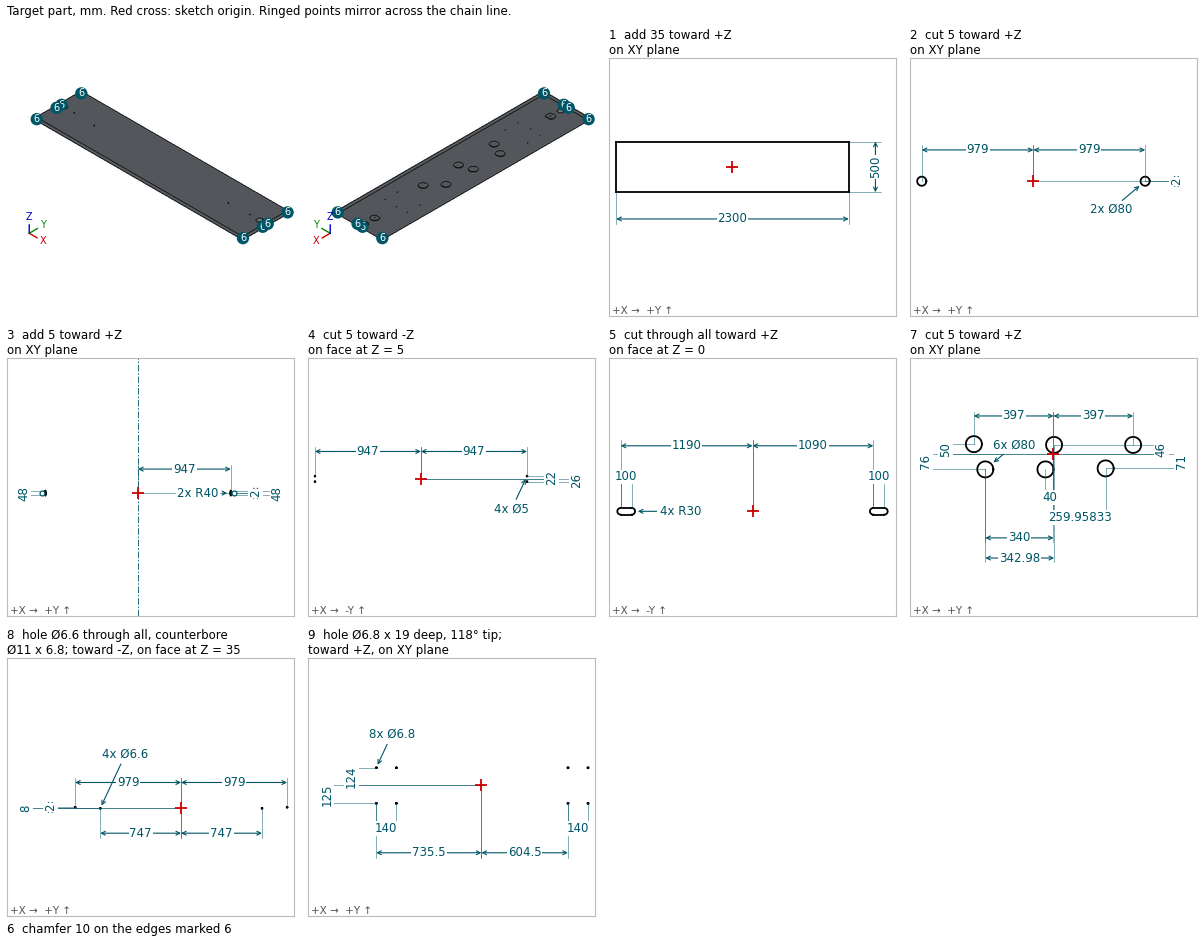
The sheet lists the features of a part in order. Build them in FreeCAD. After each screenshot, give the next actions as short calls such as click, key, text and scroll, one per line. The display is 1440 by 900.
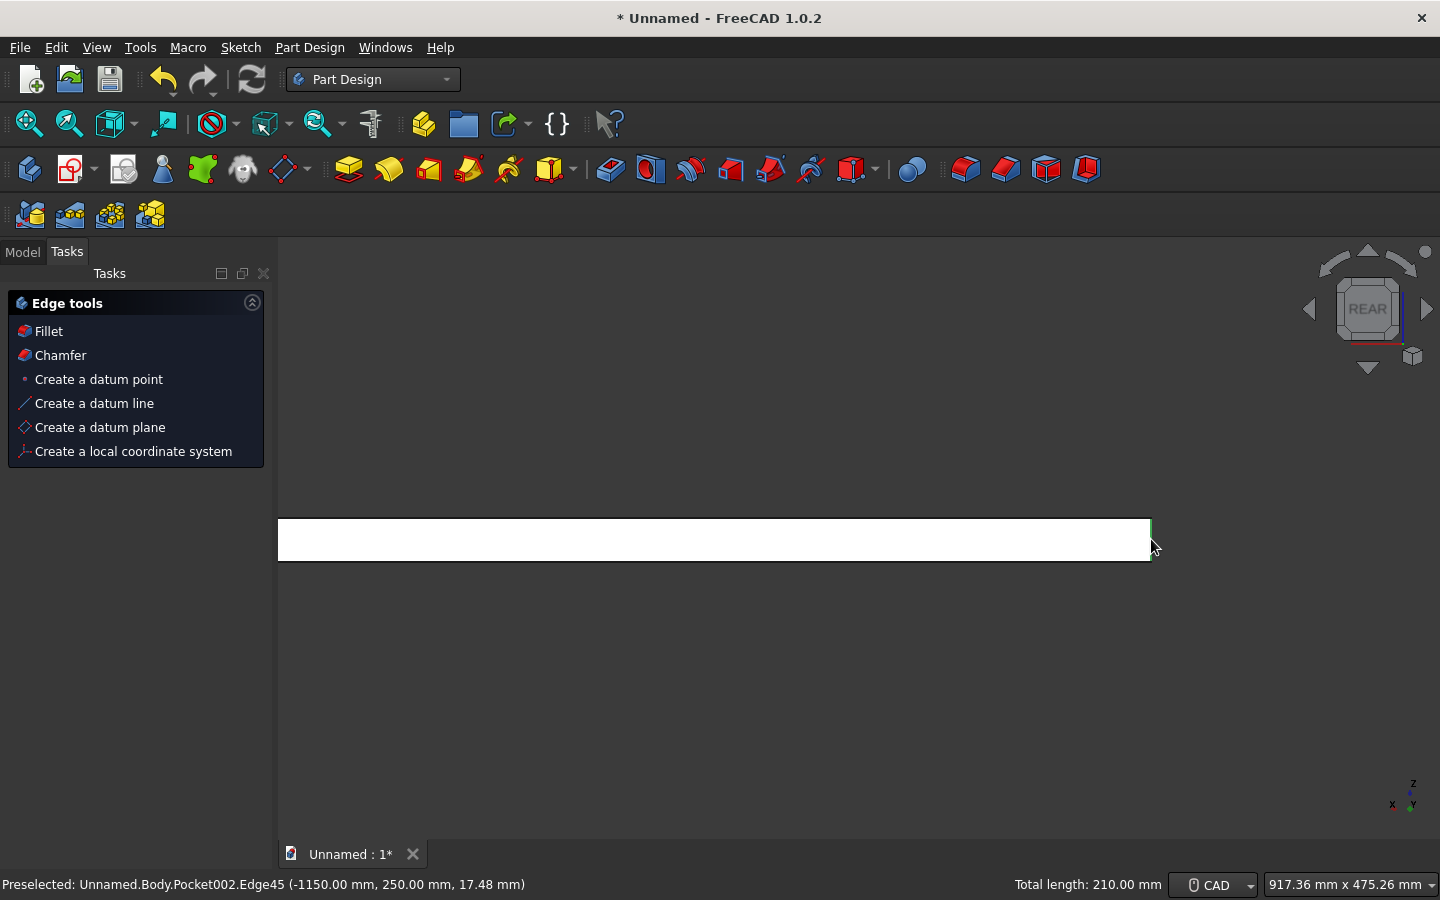
click(30, 124)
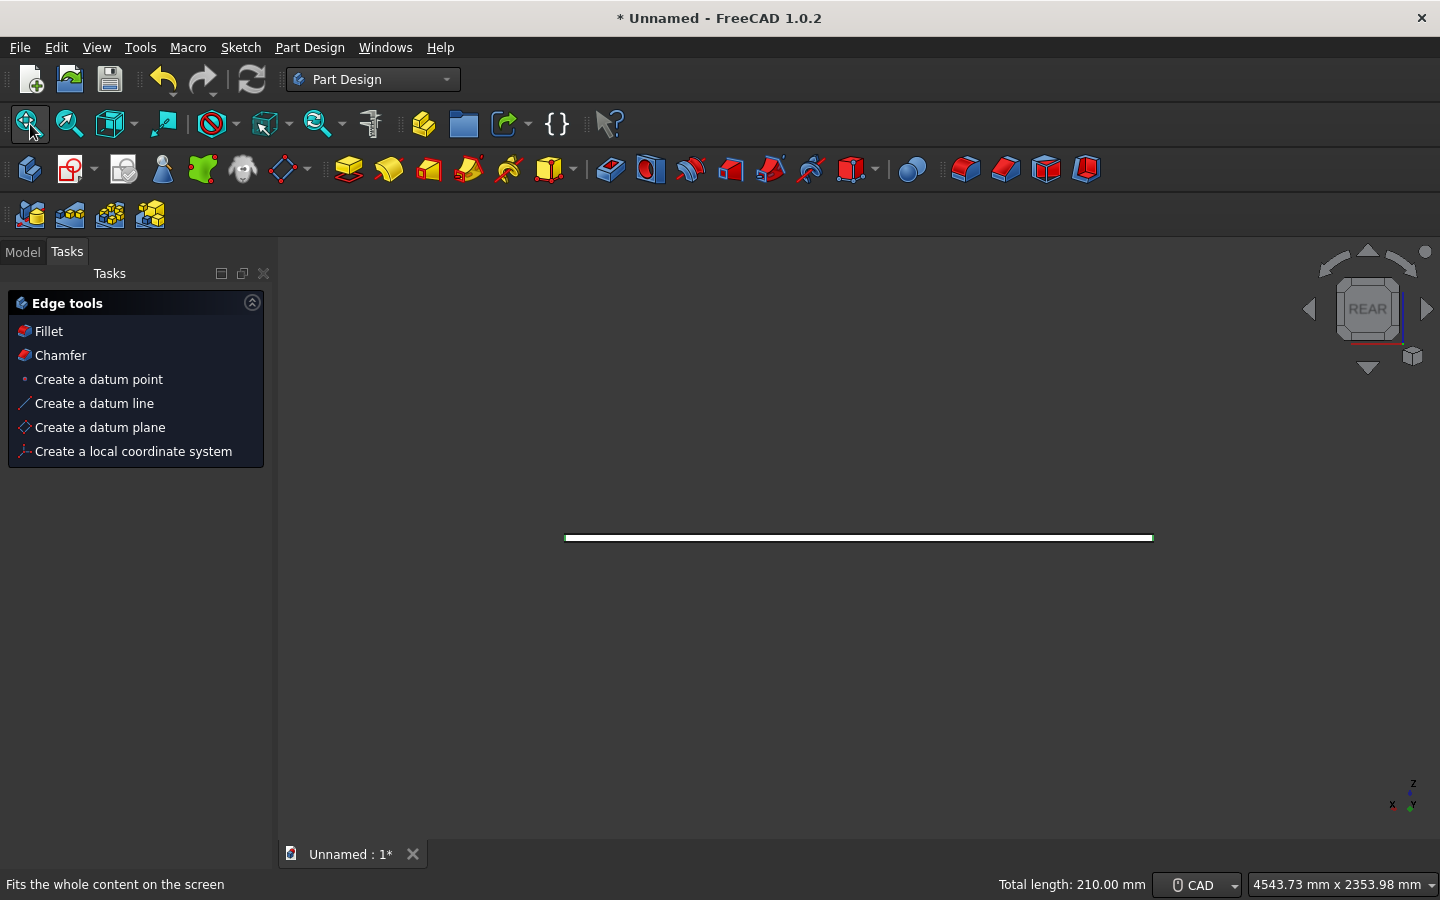
key(6)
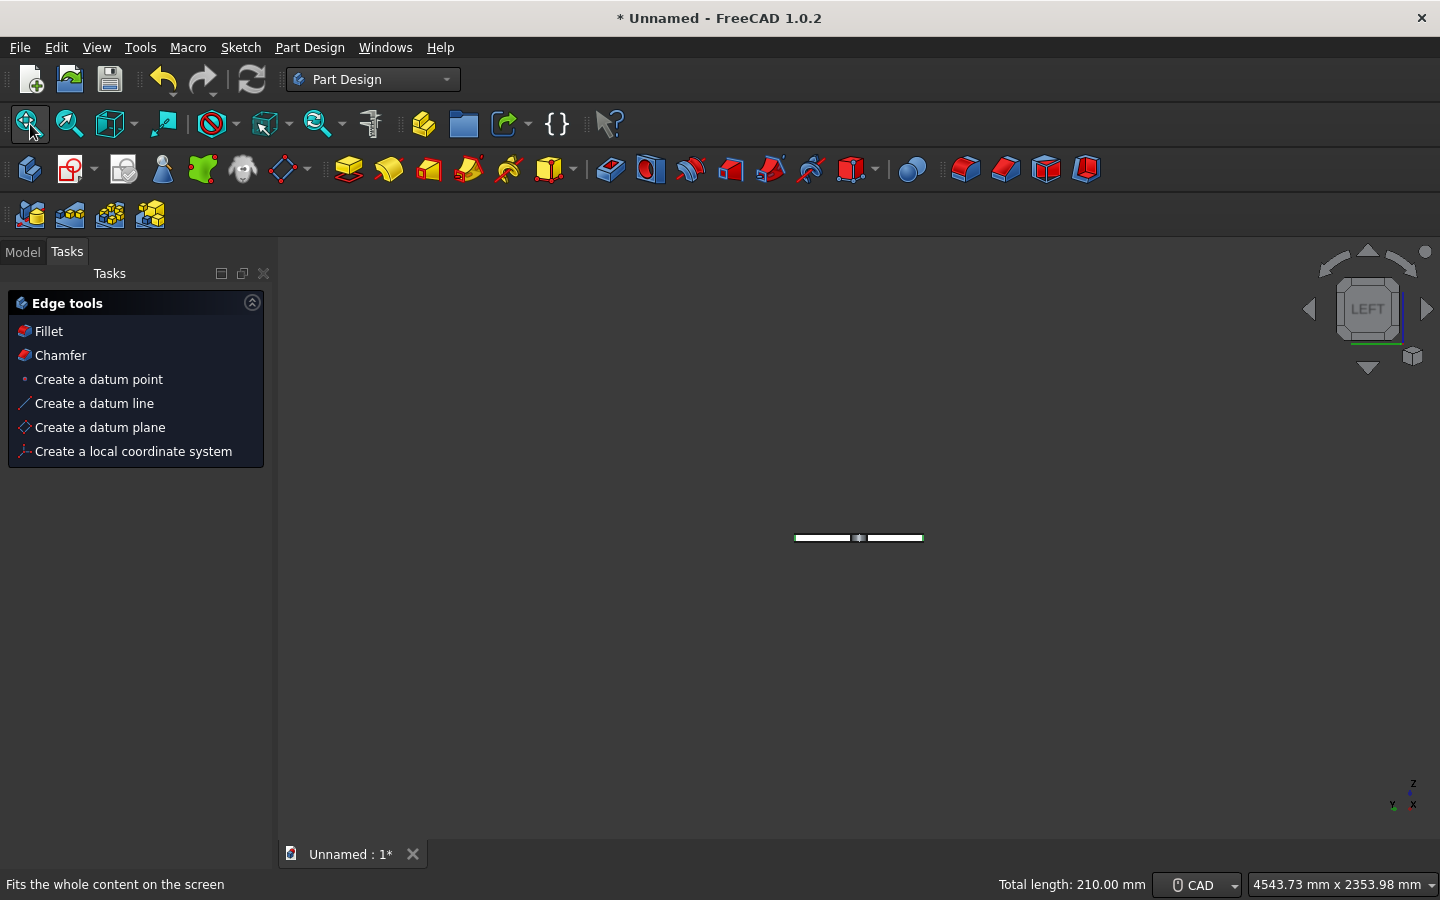
click(30, 124)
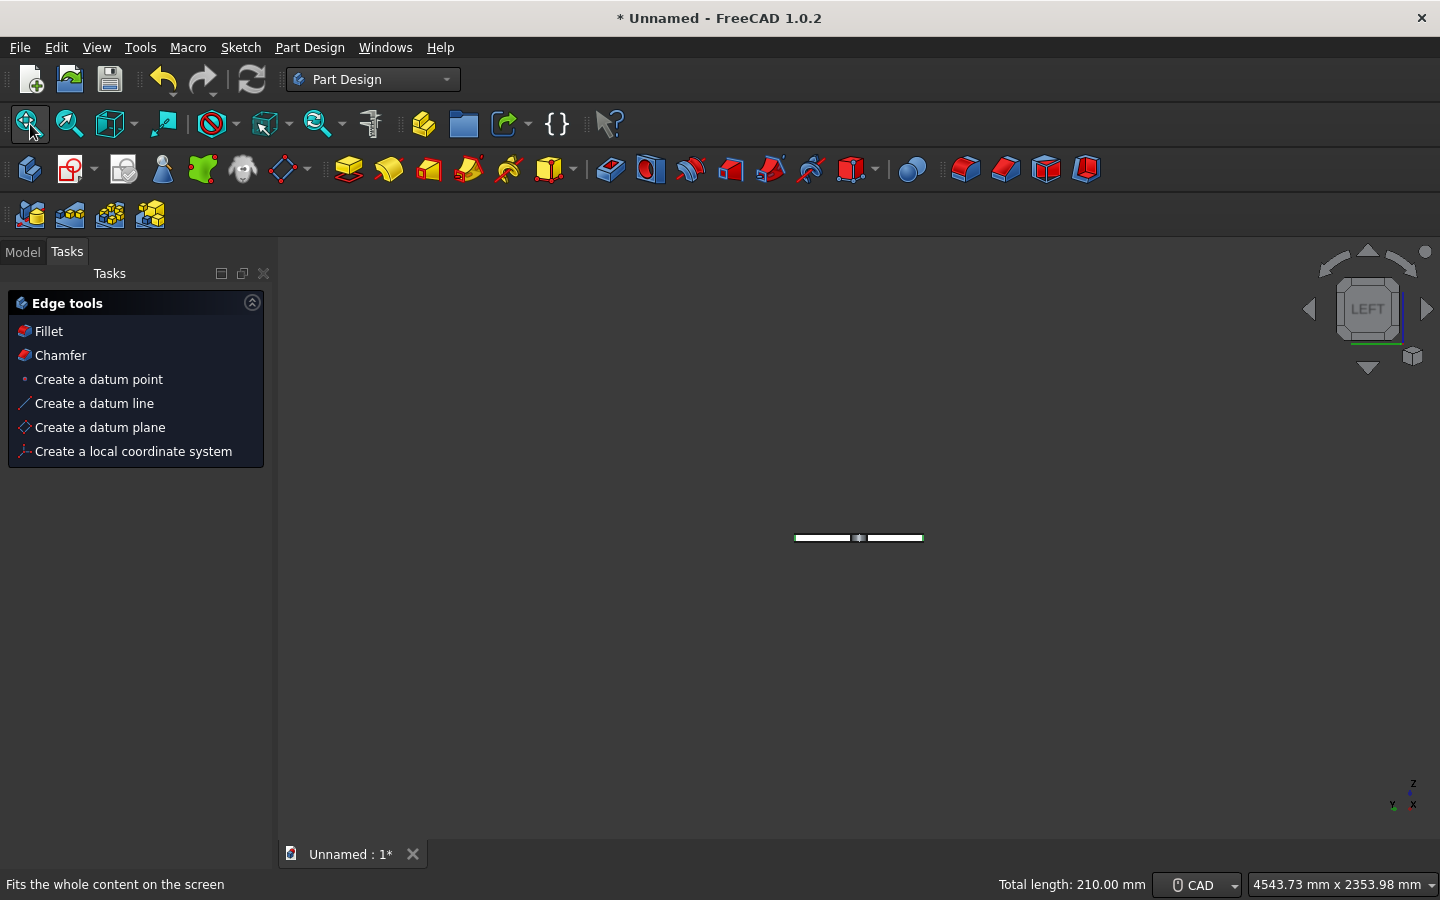
scroll(851, 537, up, 8)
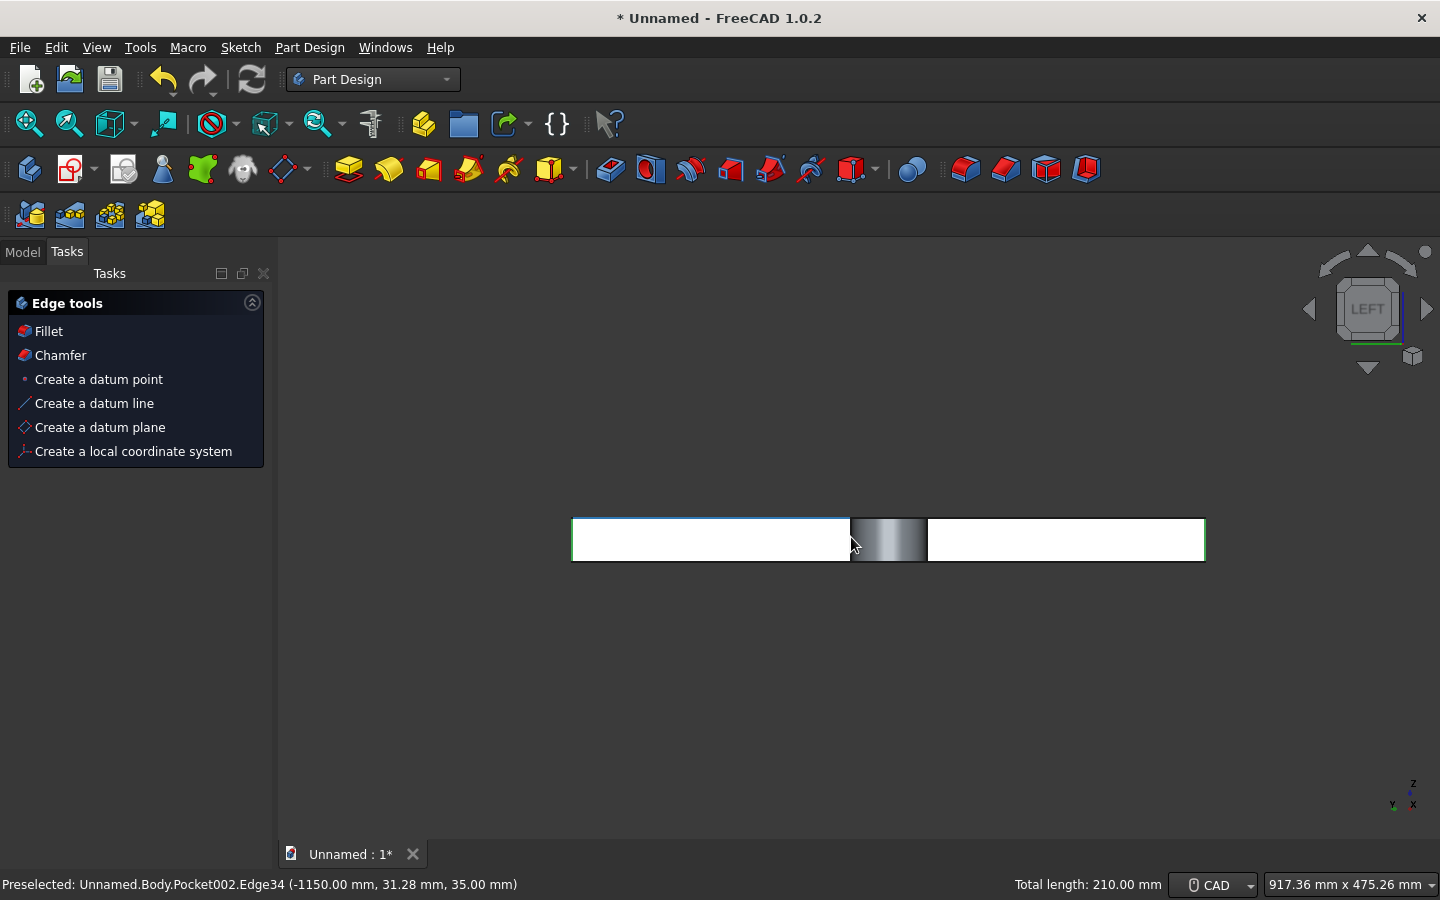
click(851, 539, ctrl)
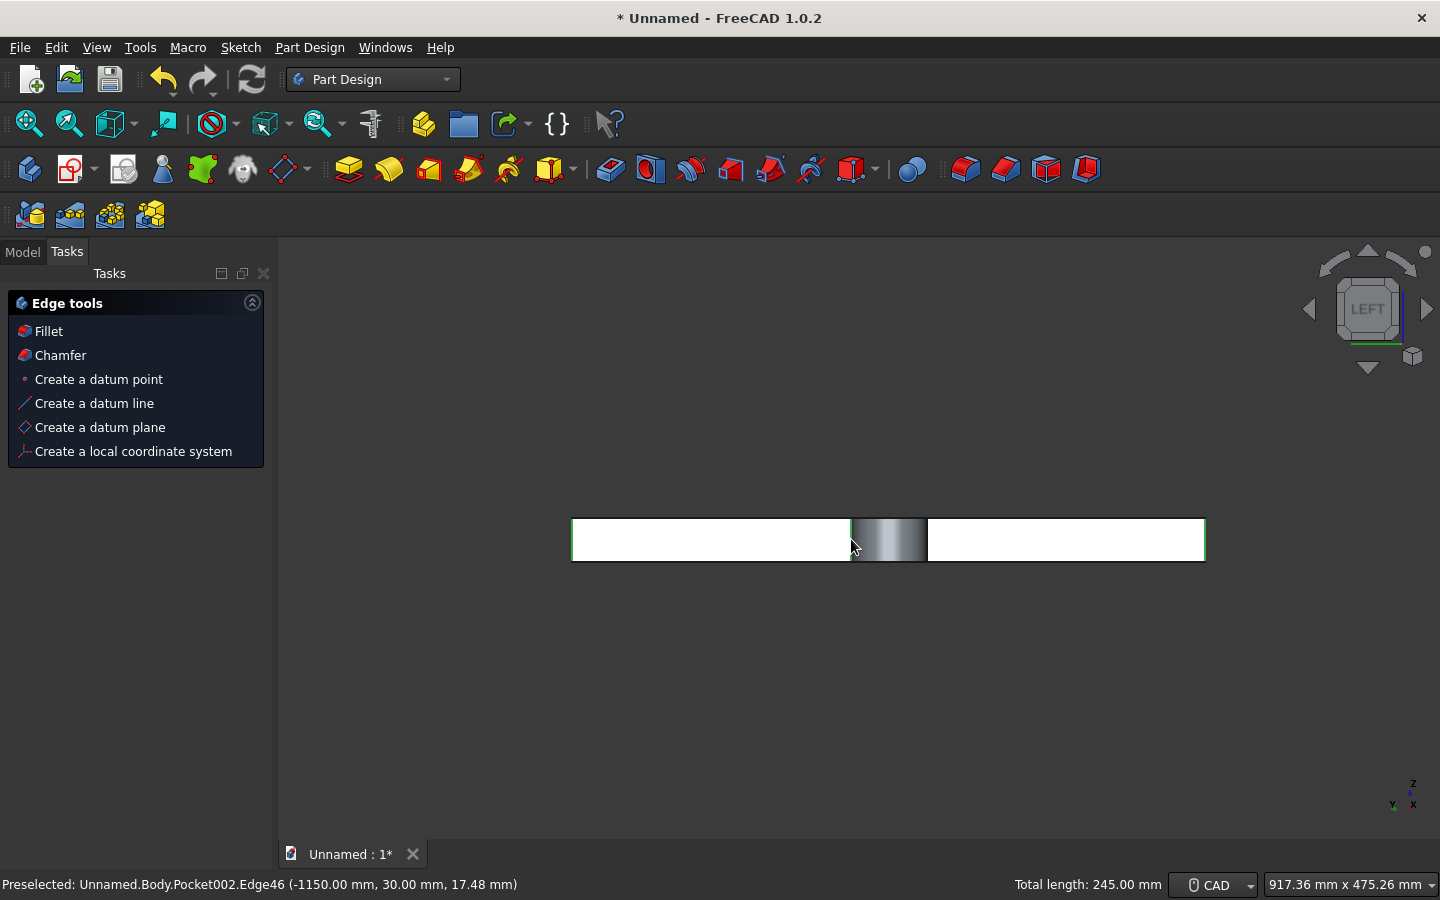
click(927, 539, ctrl)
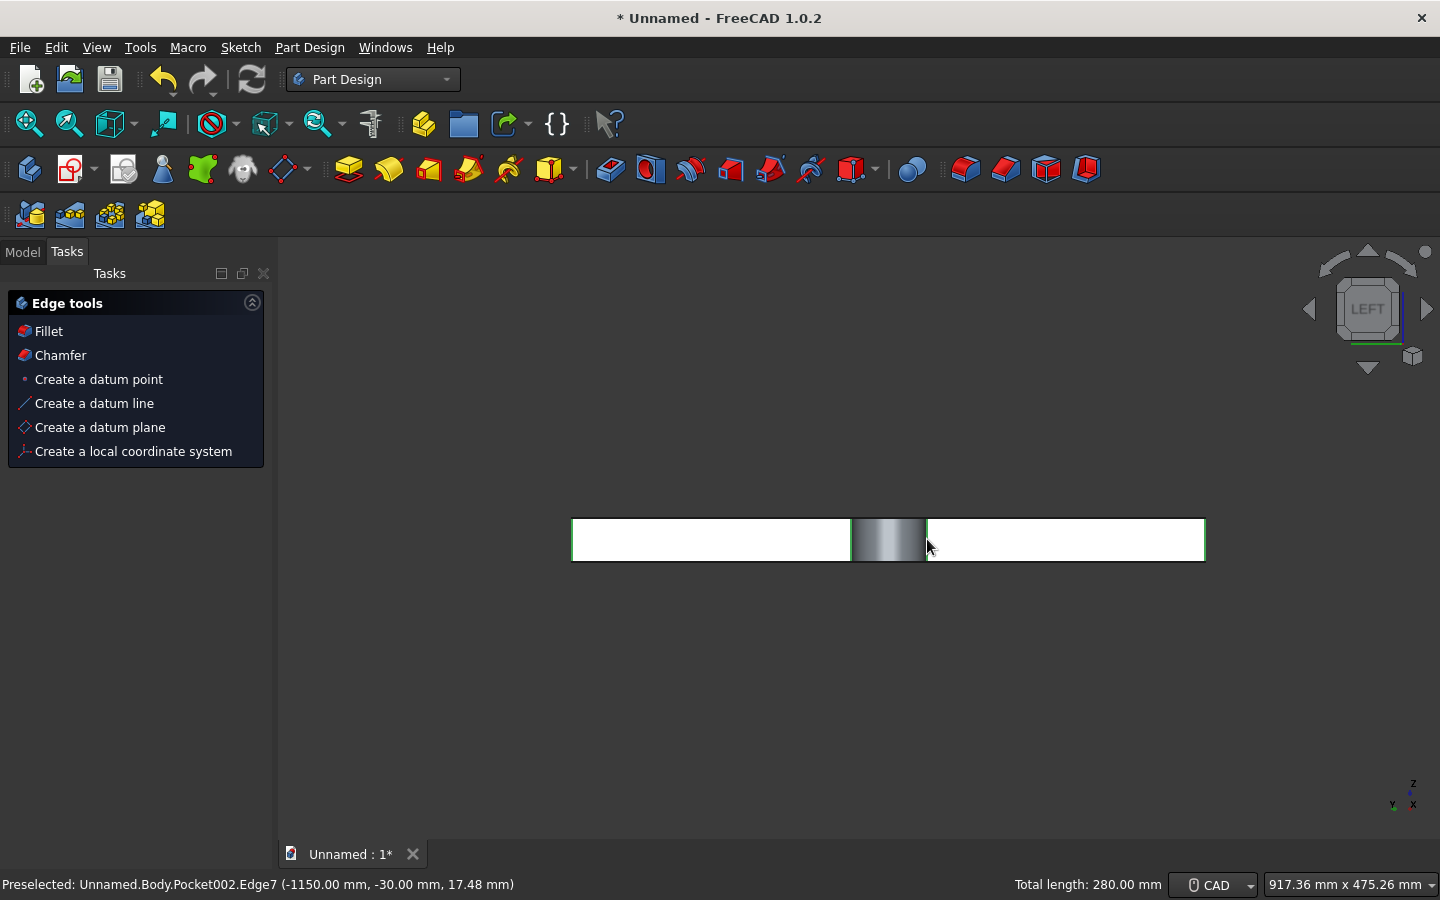
click(1006, 170)